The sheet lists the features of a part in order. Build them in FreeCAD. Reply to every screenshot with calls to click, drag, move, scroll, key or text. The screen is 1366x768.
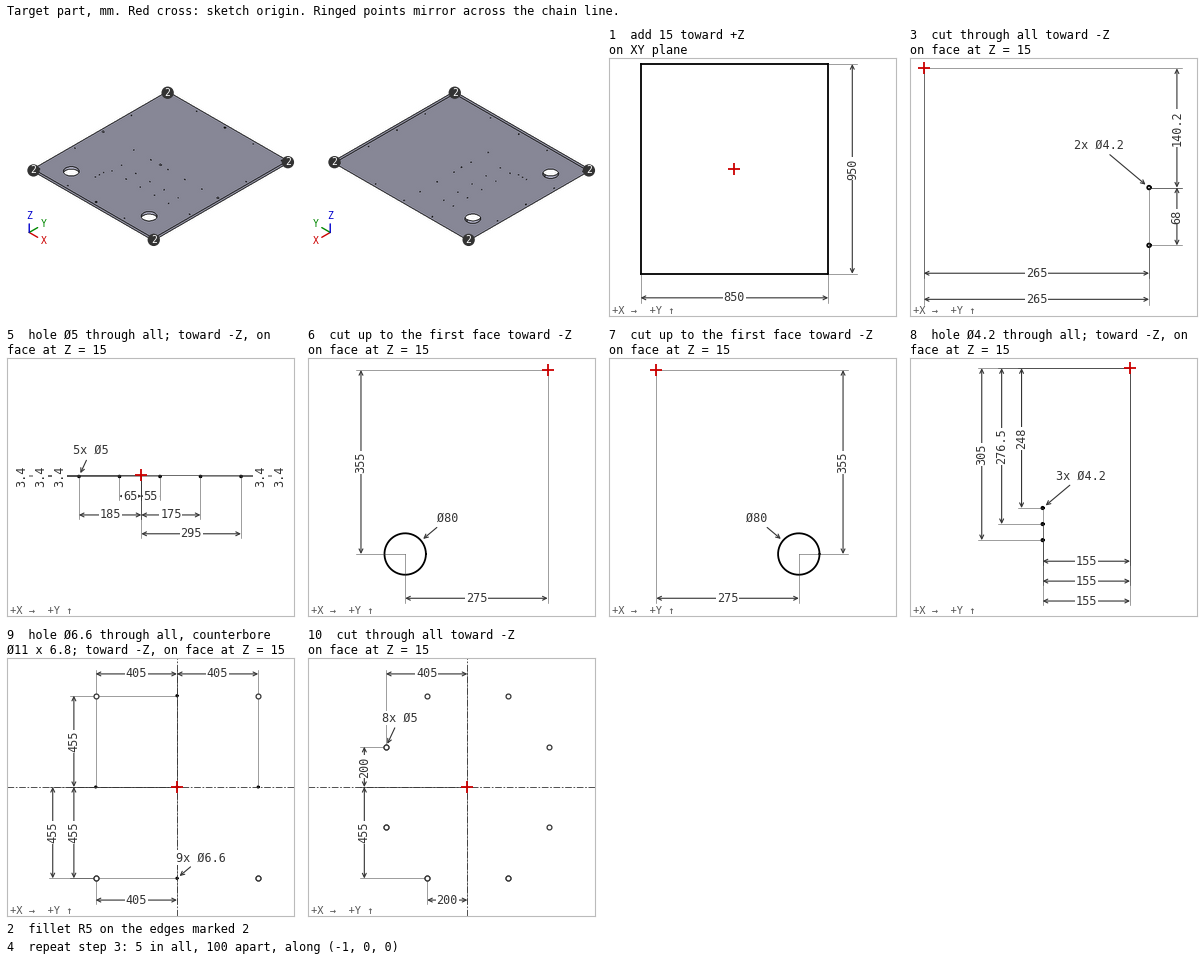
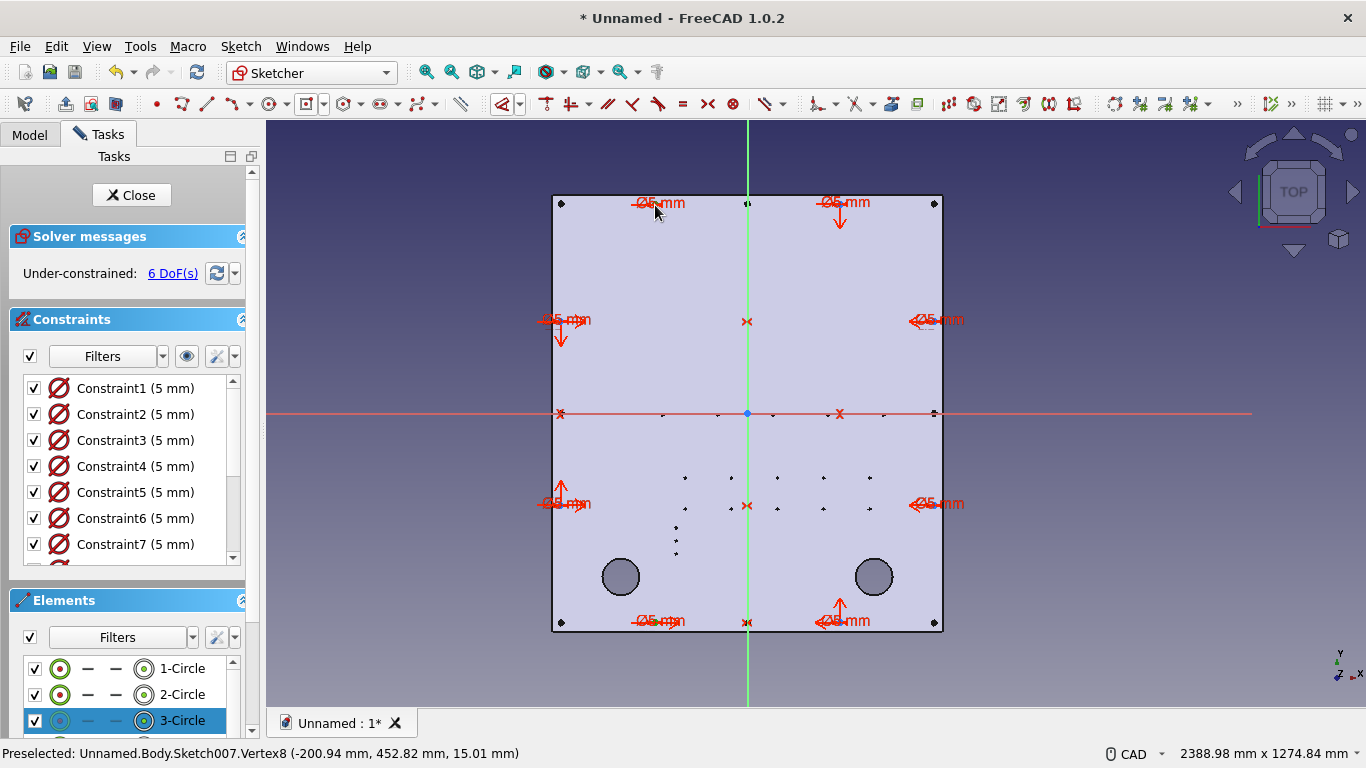
click(359, 413)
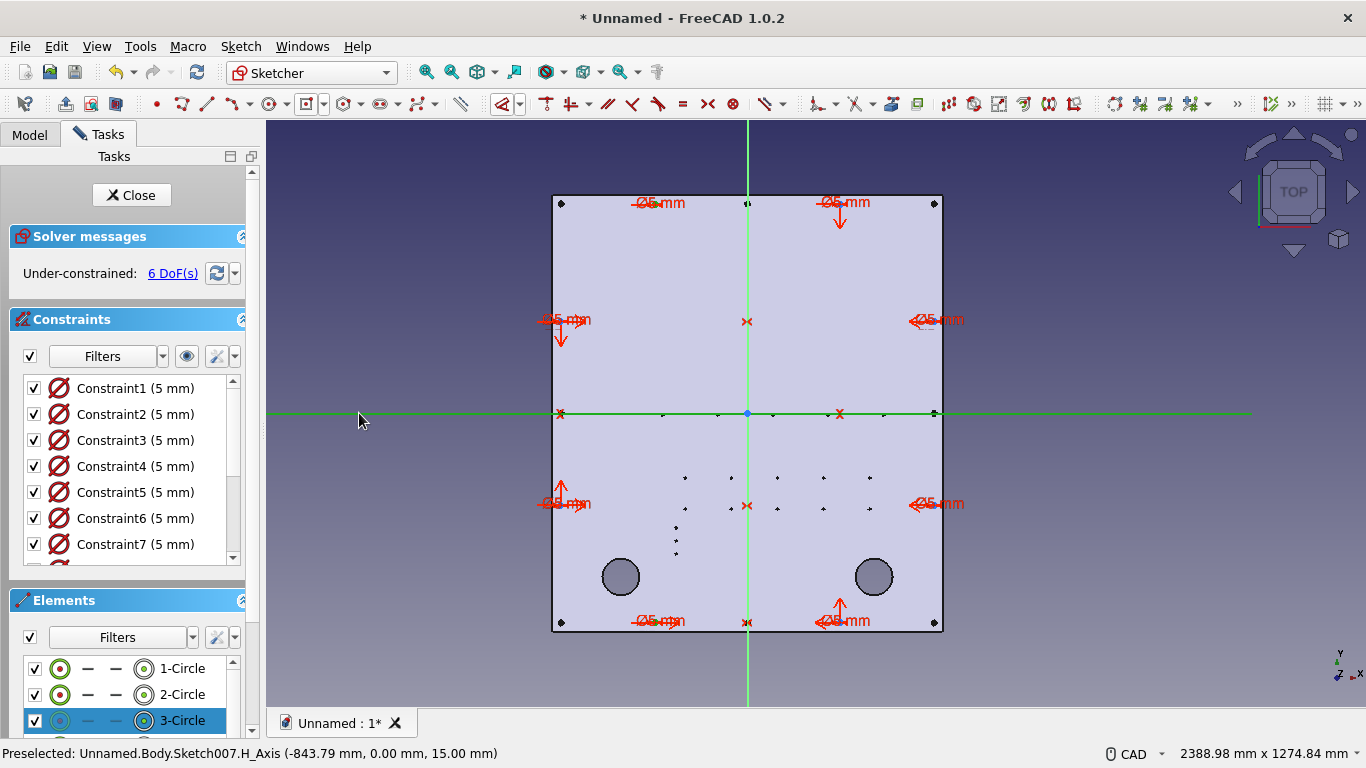
click(708, 104)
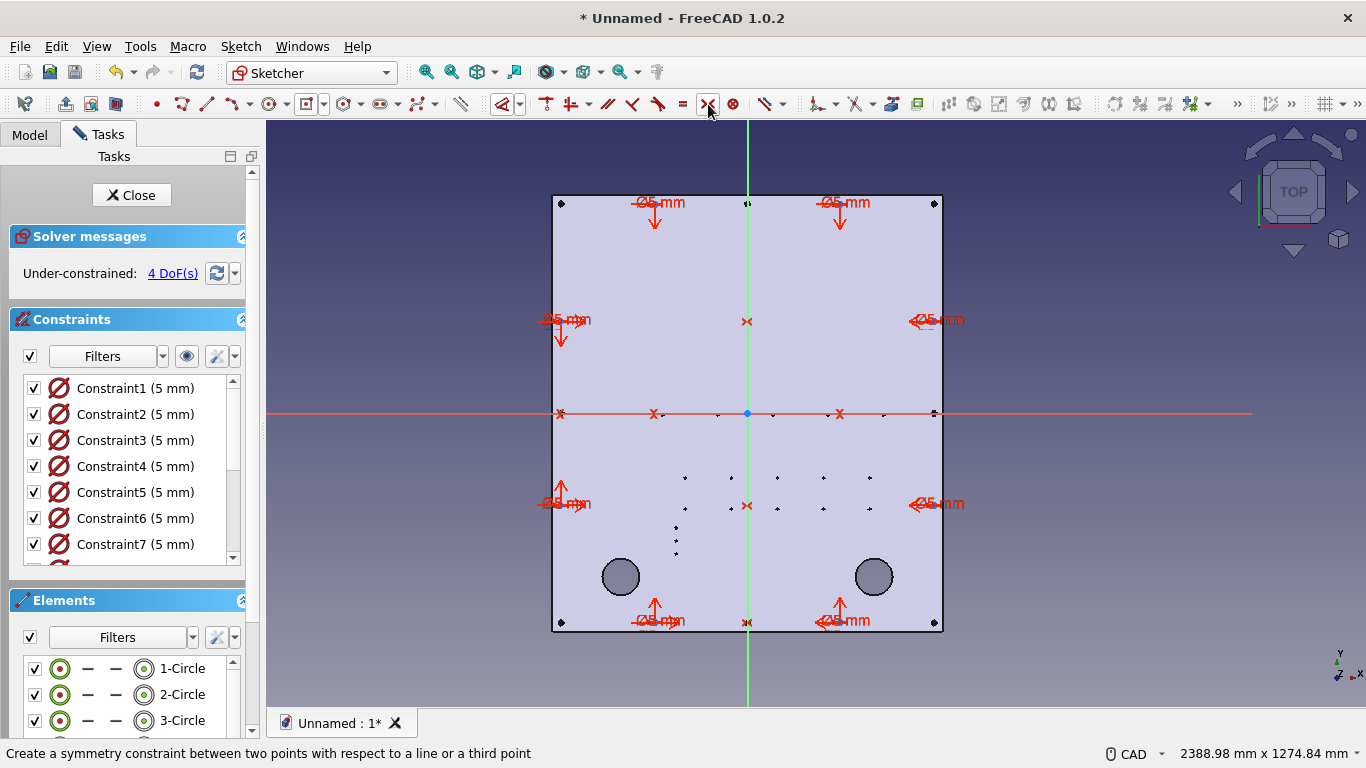
click(561, 322)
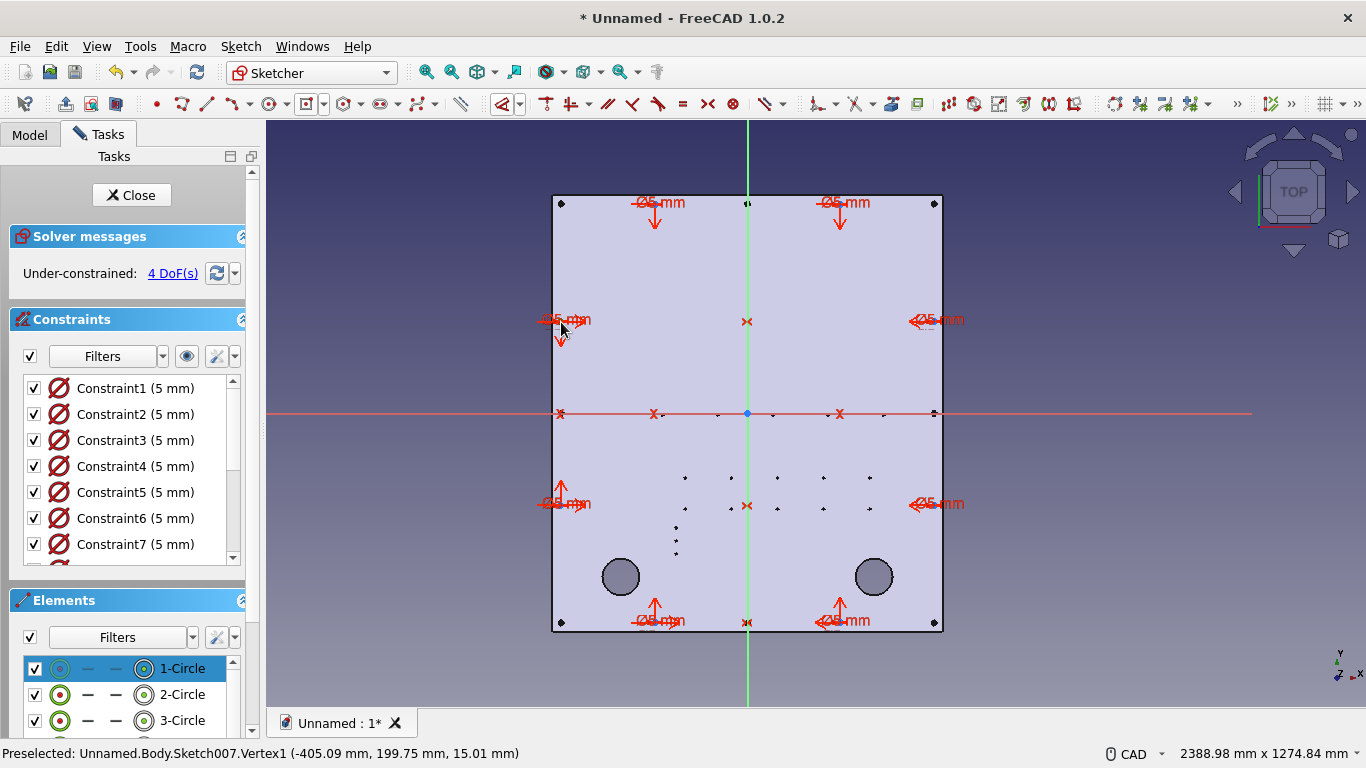
key(l)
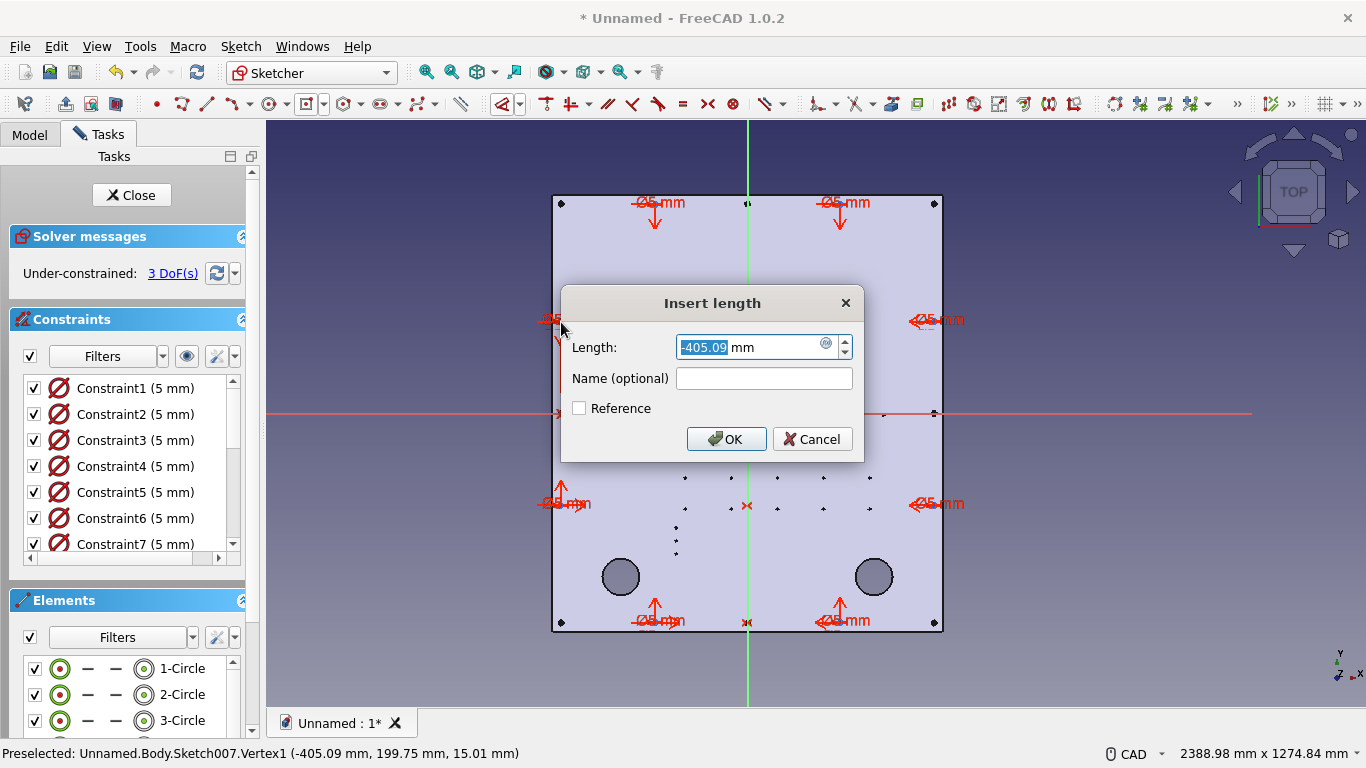
text(-405)
key(Return)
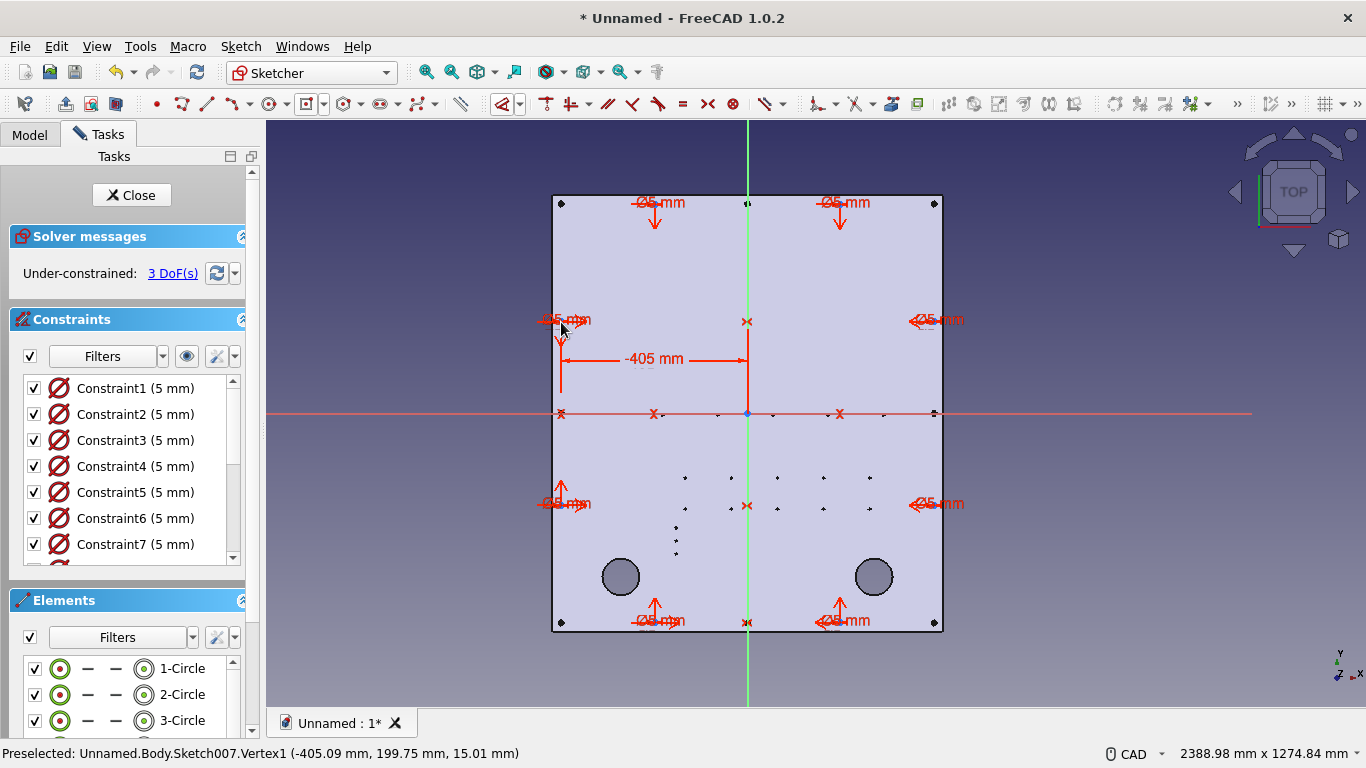
click(561, 322)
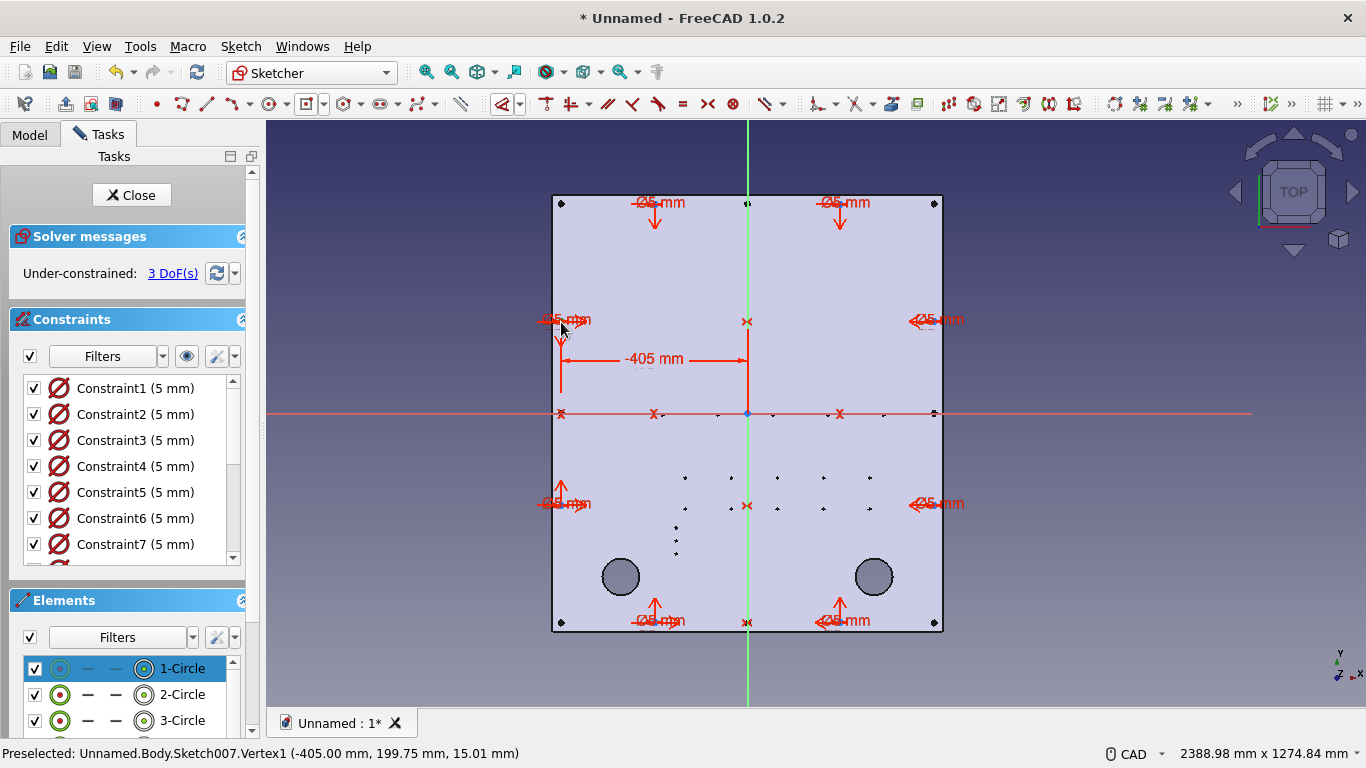
key(i)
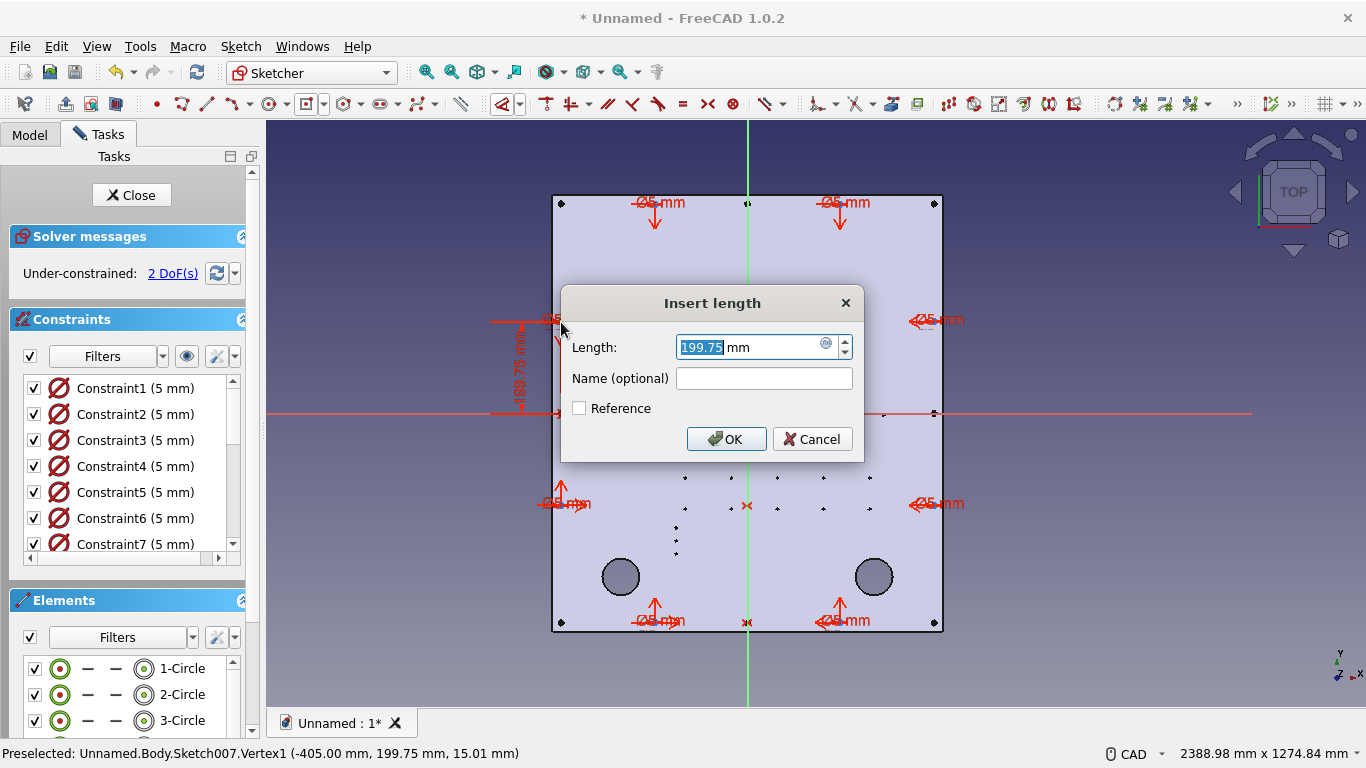
text(200)
key(Return)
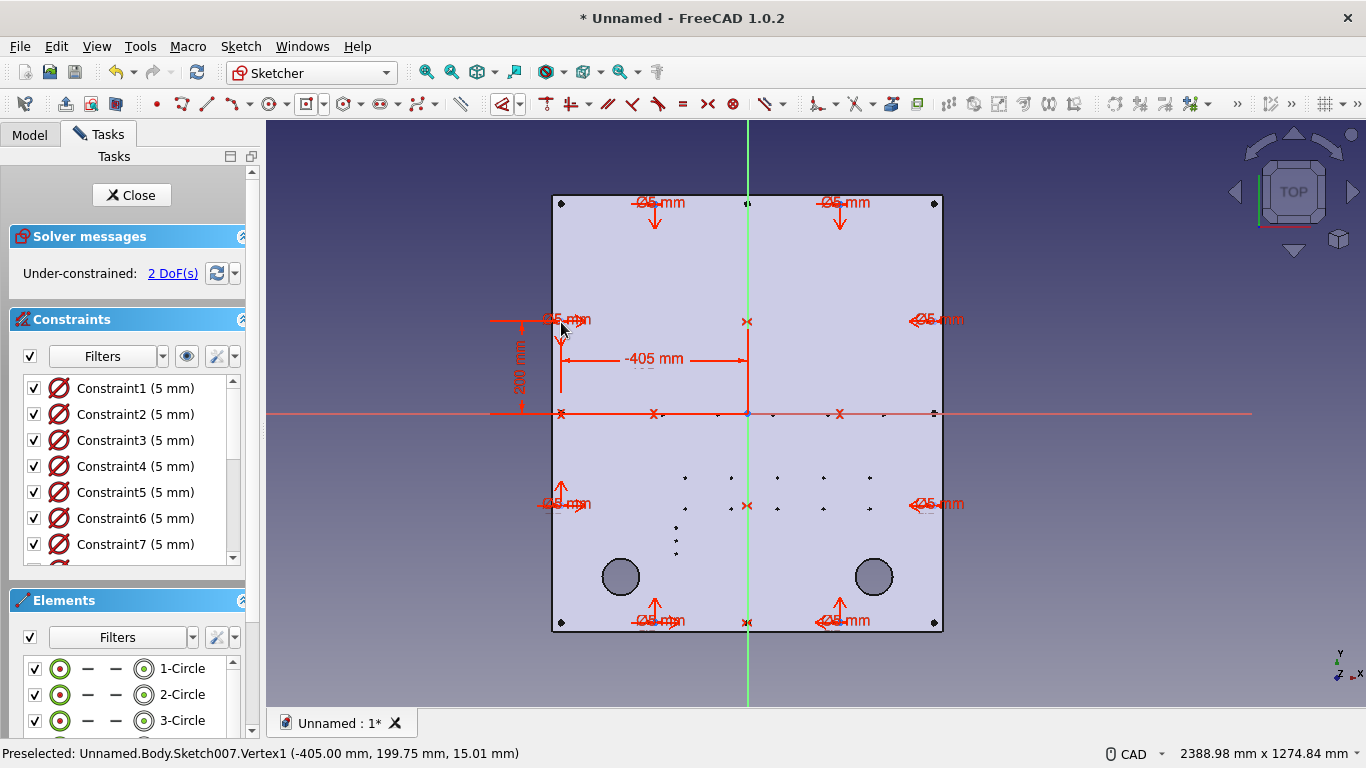
click(655, 623)